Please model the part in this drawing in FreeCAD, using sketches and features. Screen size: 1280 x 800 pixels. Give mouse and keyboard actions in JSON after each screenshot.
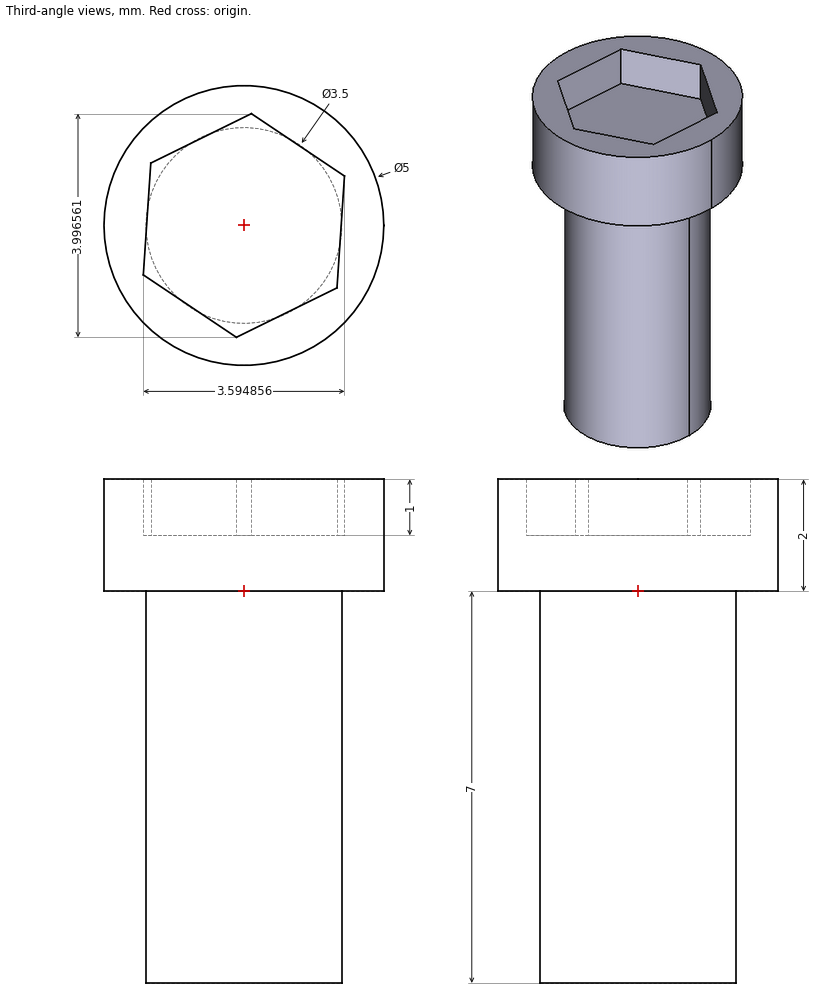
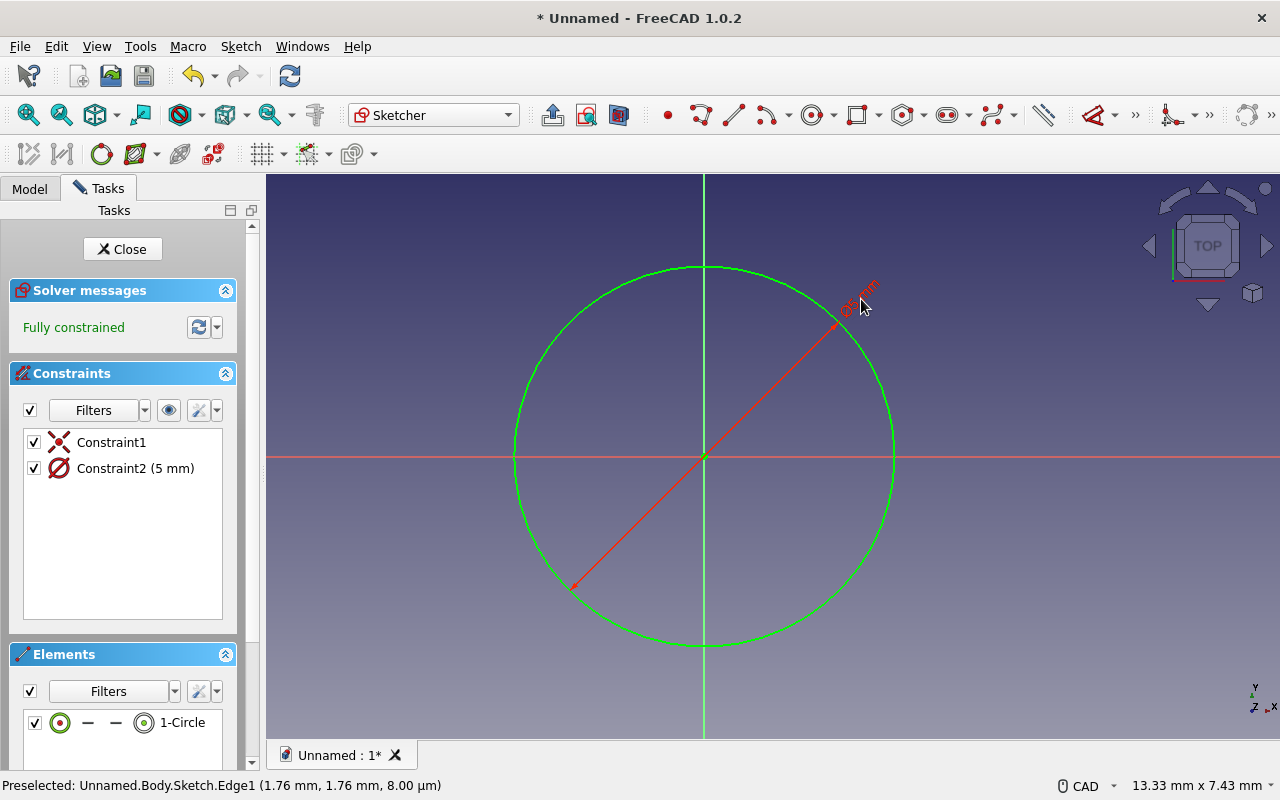
{"action": "left_click", "coordinate": [123, 249]}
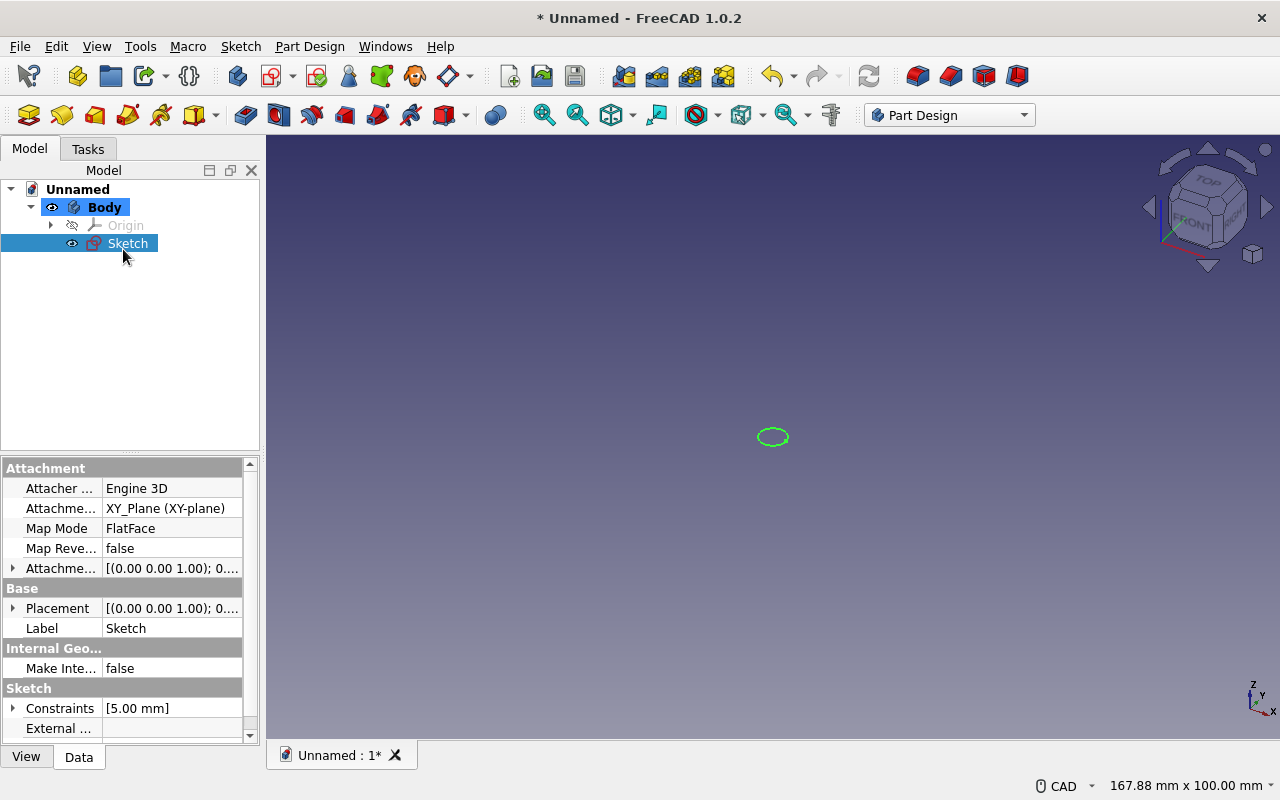
{"action": "left_click", "coordinate": [29, 116]}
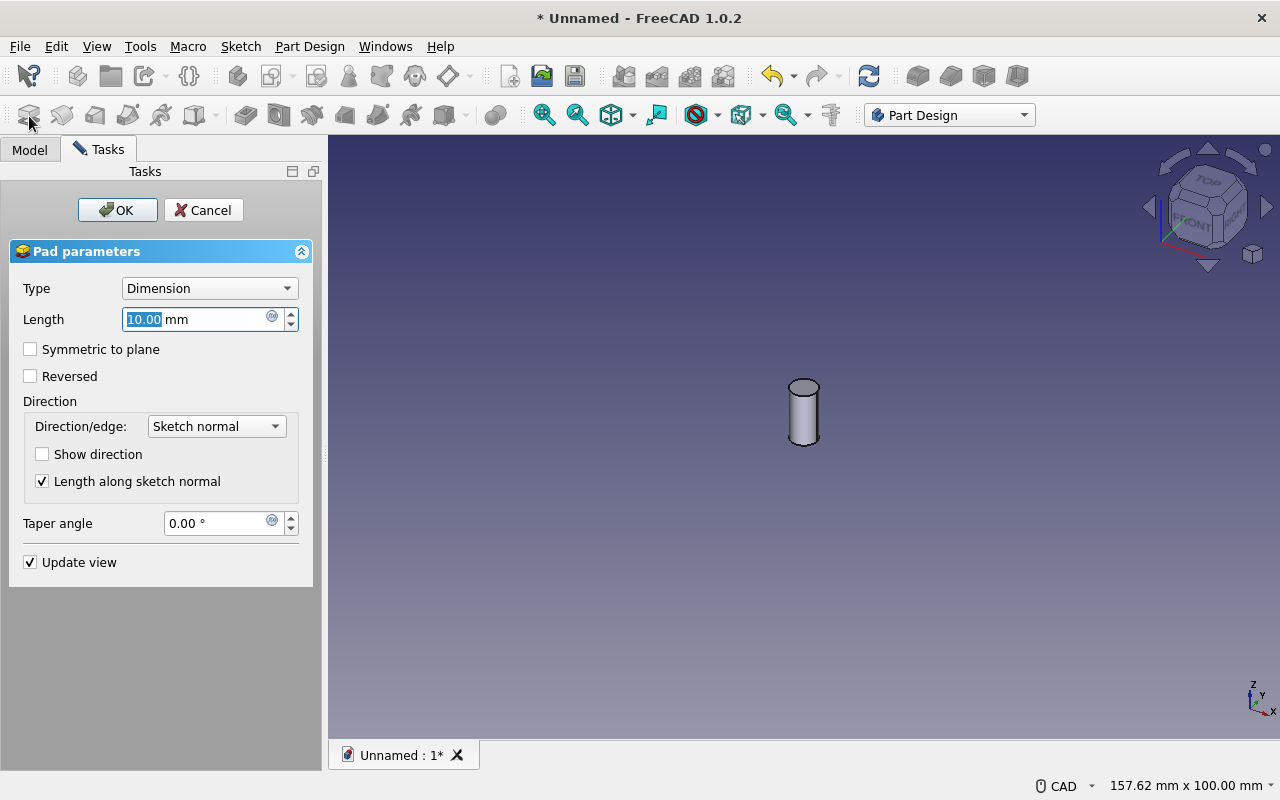
{"action": "type", "text": "2"}
{"action": "key", "text": "Tab"}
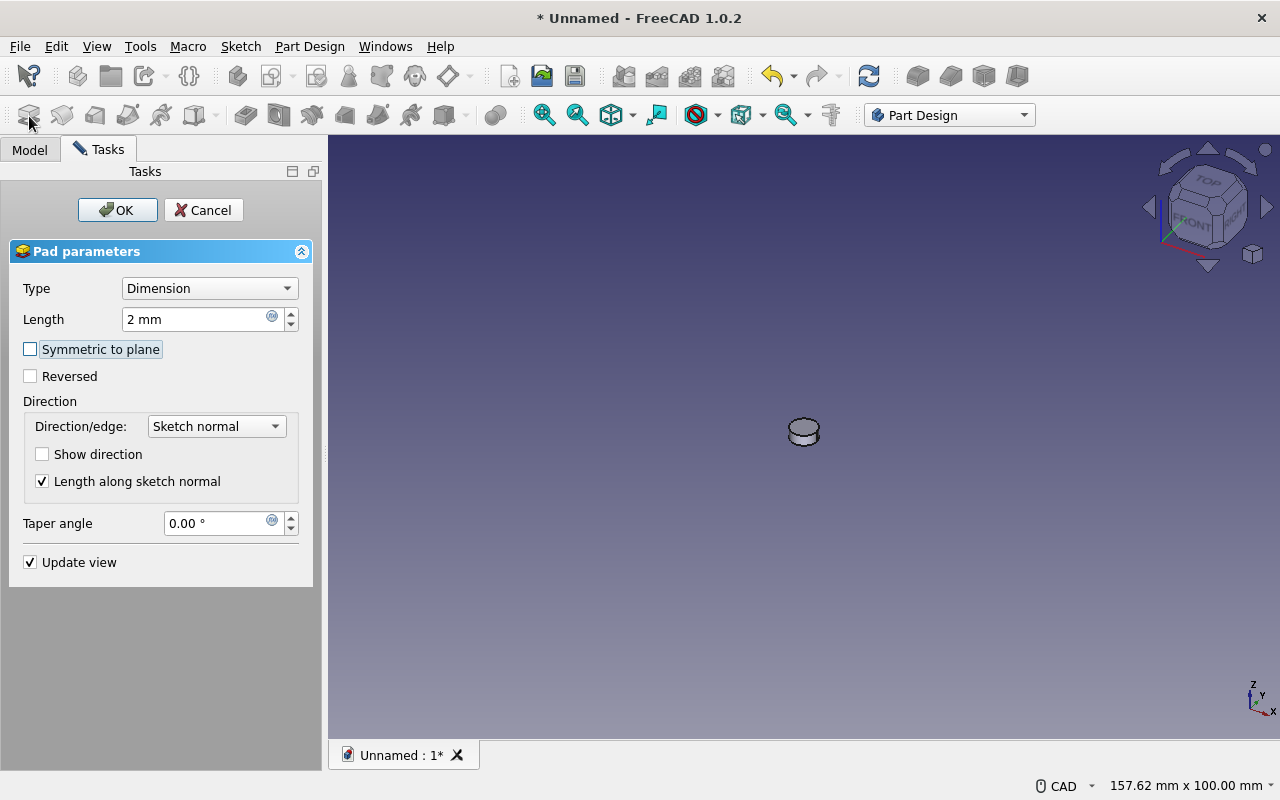
{"action": "left_click", "coordinate": [118, 210]}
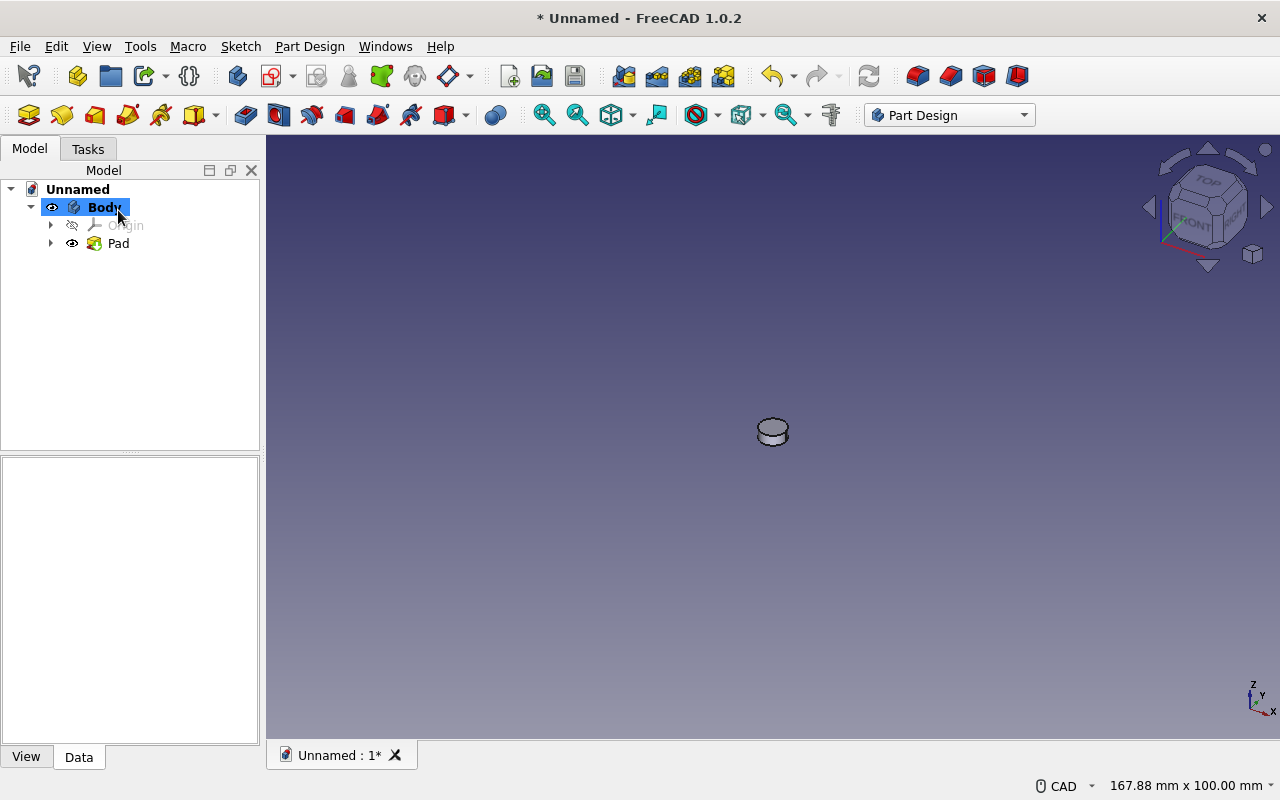
{"action": "left_click", "coordinate": [545, 116]}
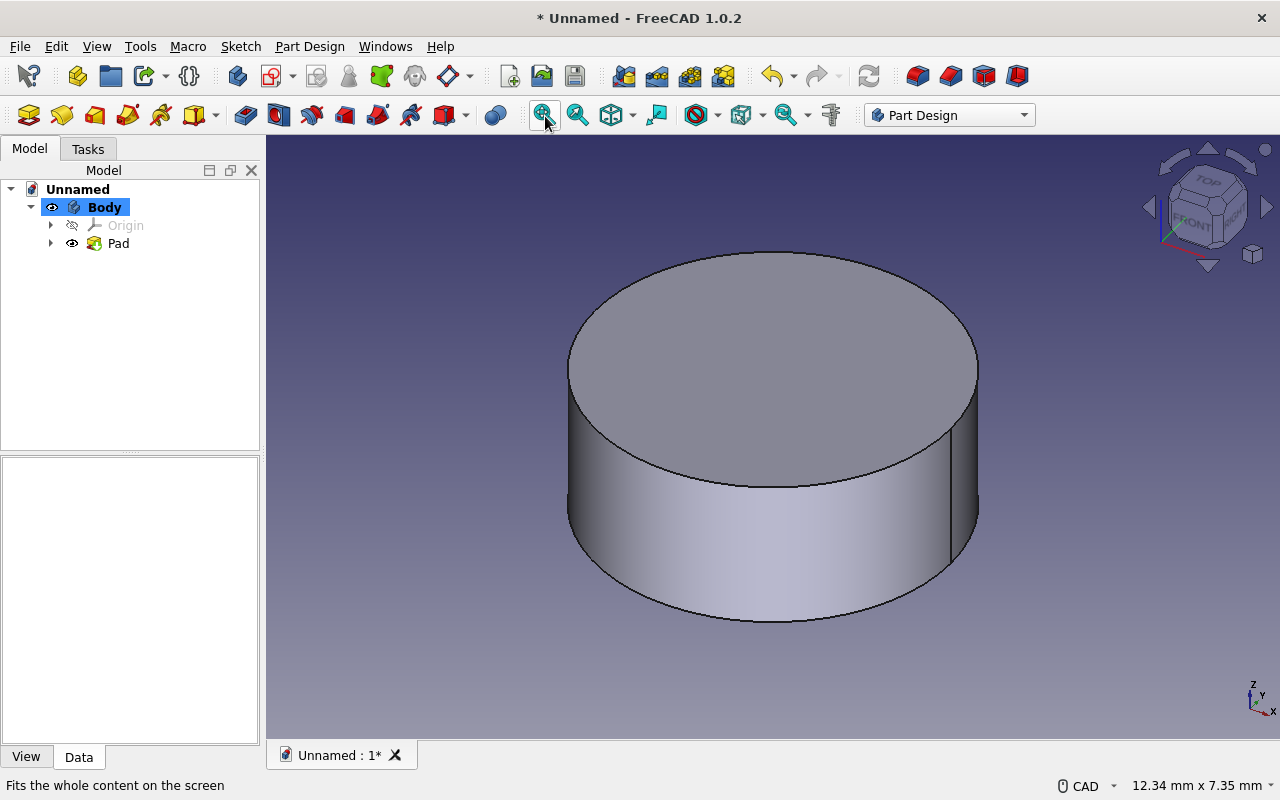
{"action": "left_click", "coordinate": [773, 369]}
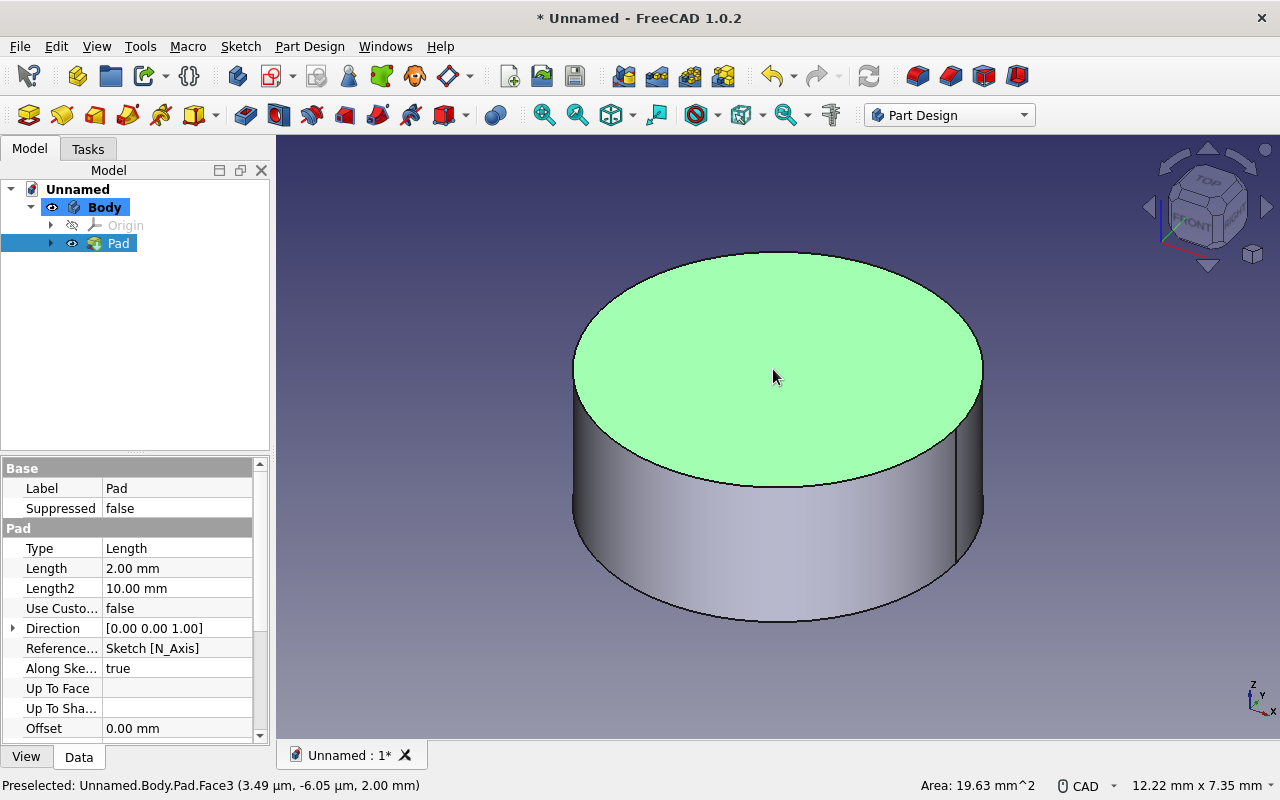
{"action": "left_click", "coordinate": [270, 76]}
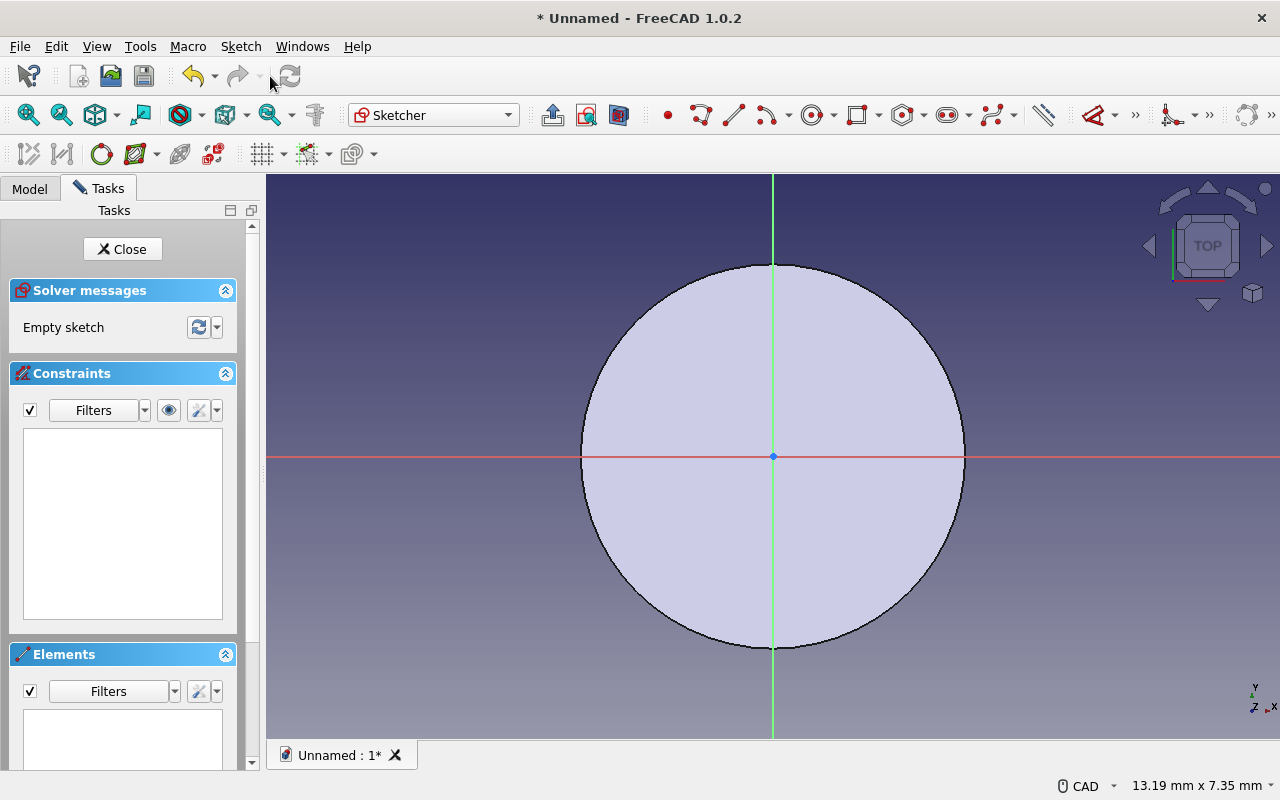
{"action": "left_click", "coordinate": [902, 116]}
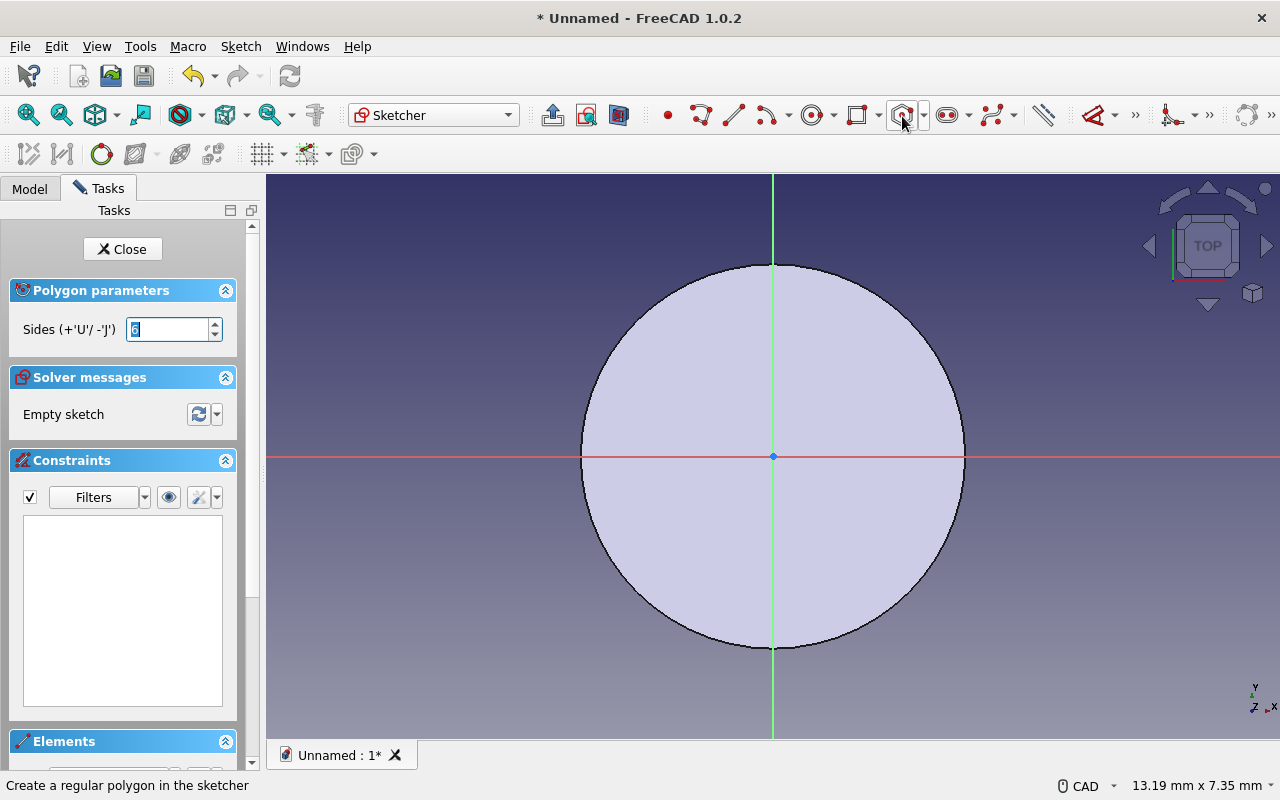
{"action": "left_click", "coordinate": [773, 456]}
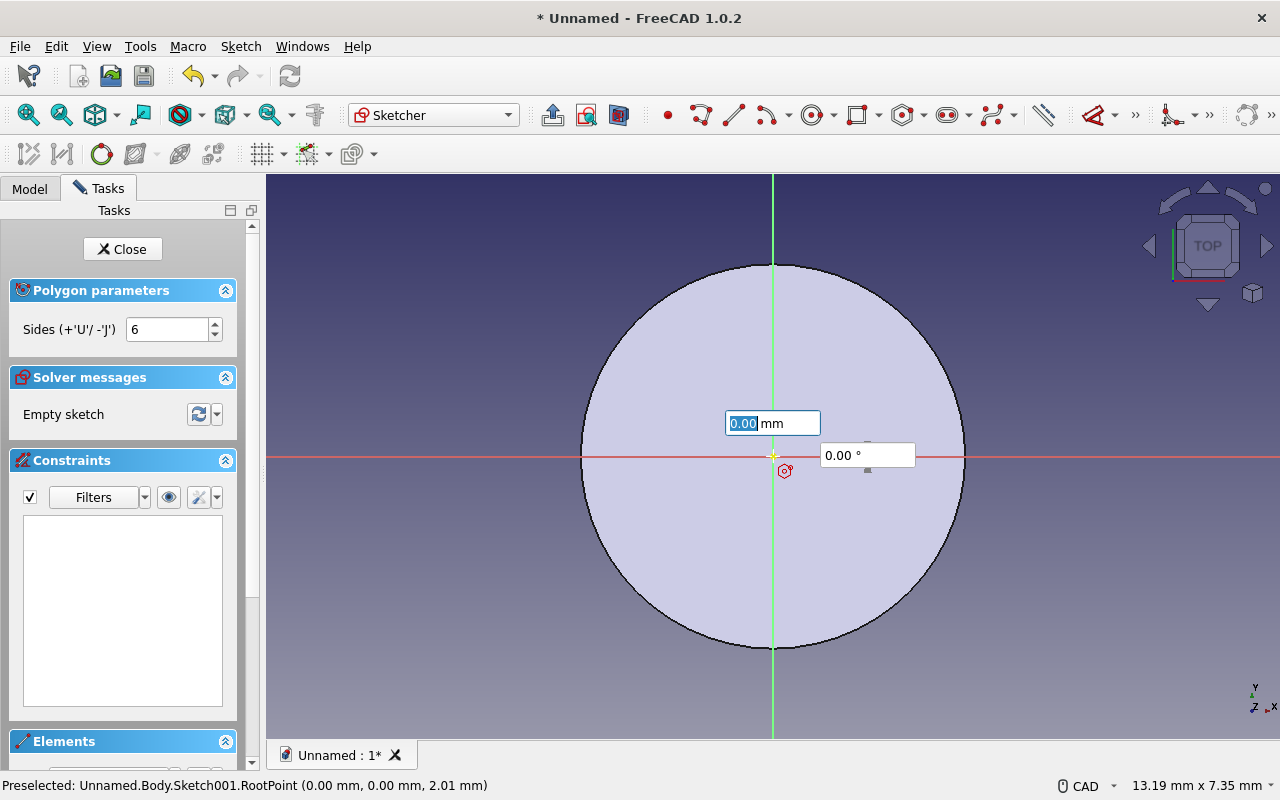
{"action": "left_click", "coordinate": [901, 542]}
{"action": "right_click", "coordinate": [901, 542]}